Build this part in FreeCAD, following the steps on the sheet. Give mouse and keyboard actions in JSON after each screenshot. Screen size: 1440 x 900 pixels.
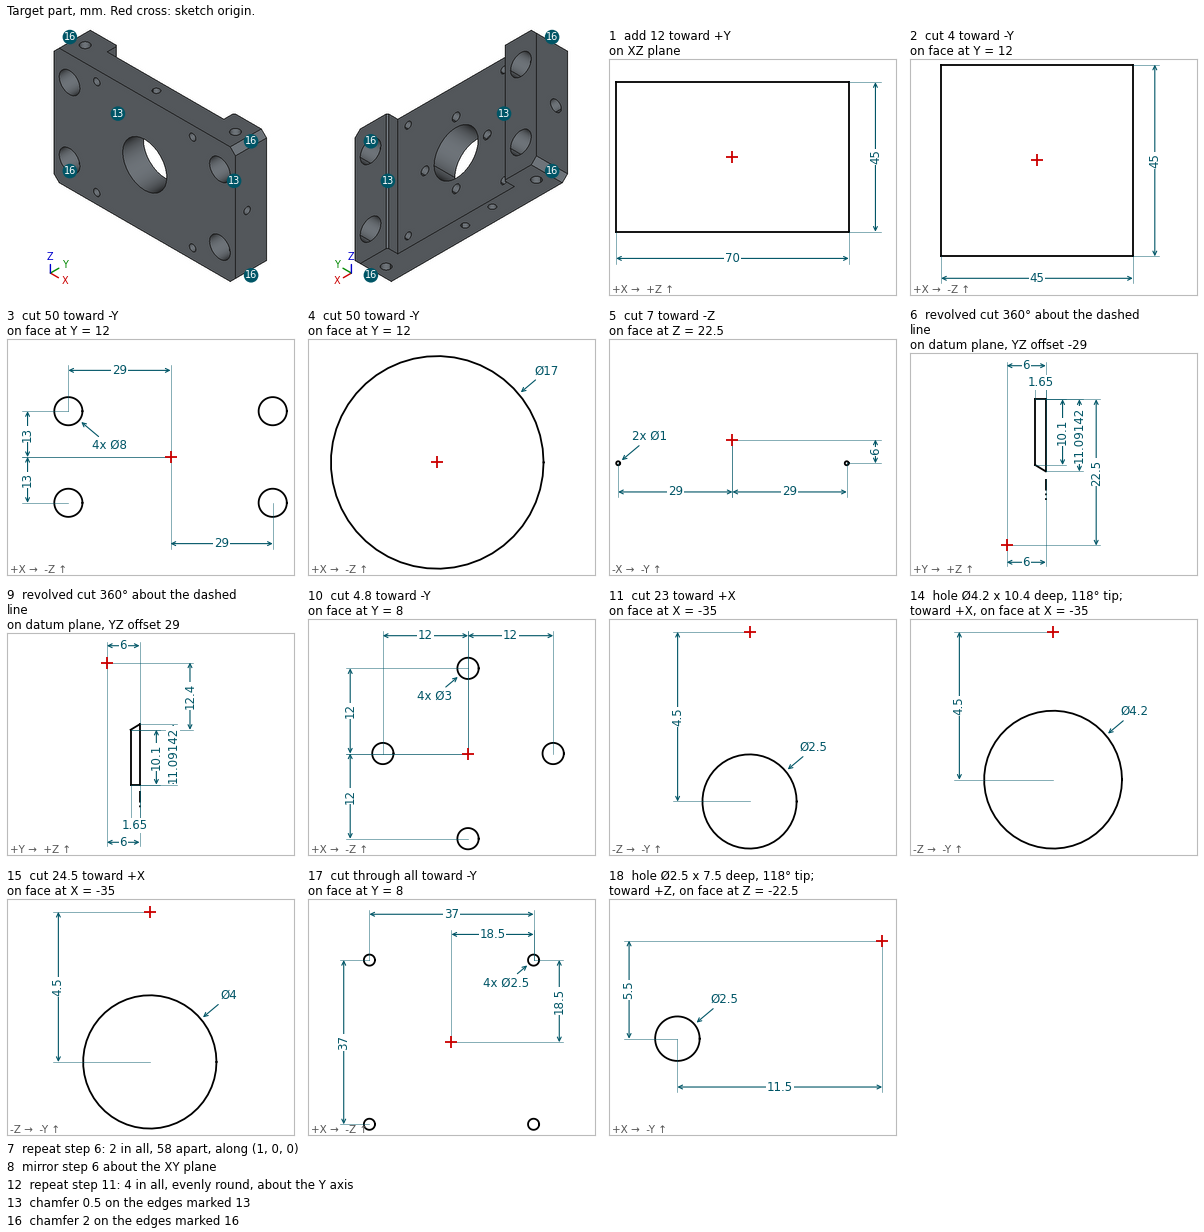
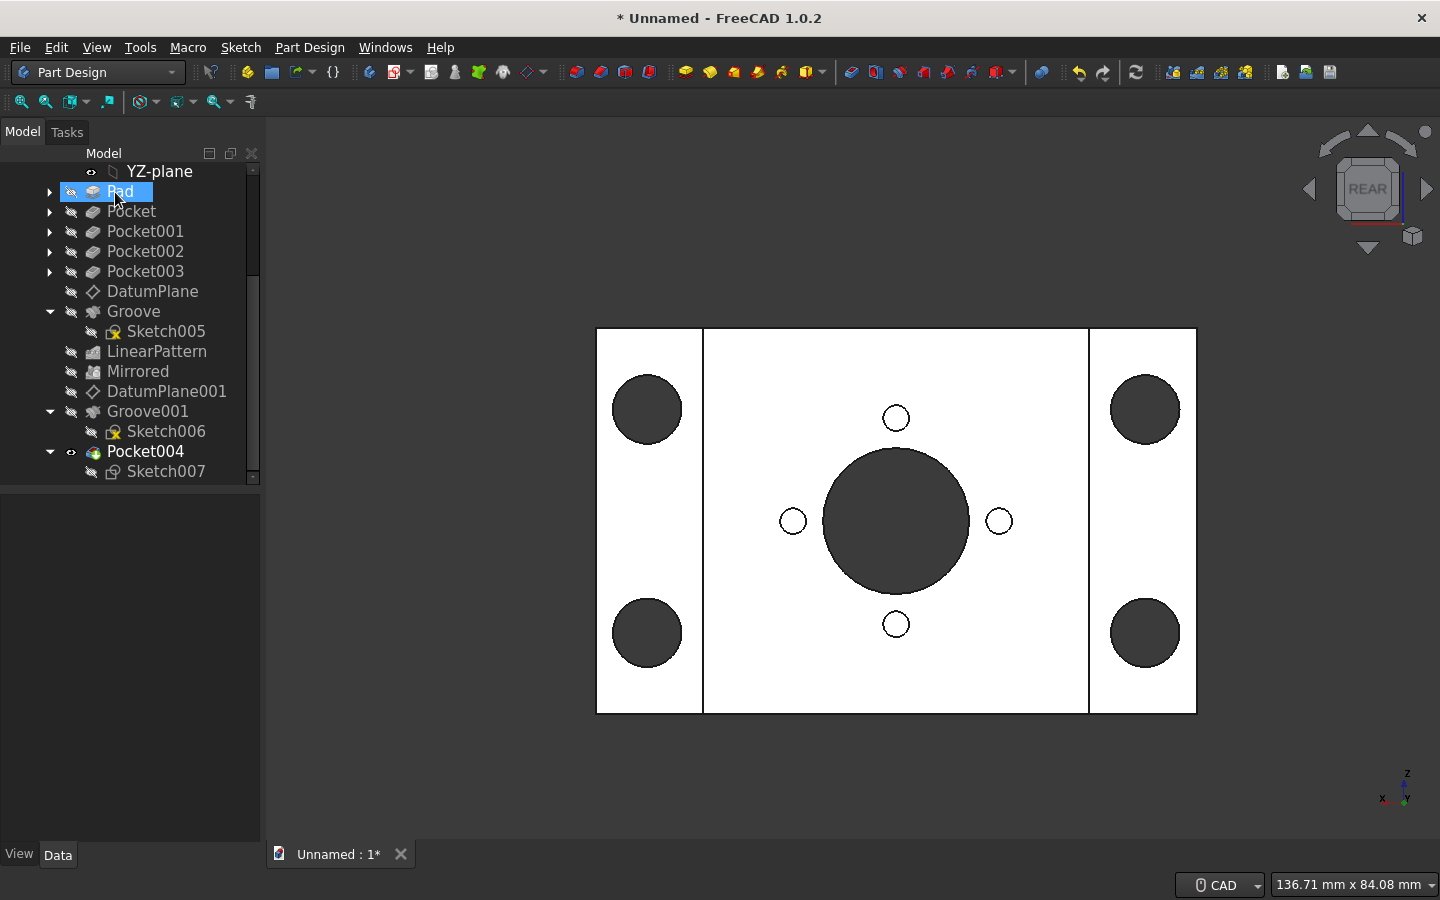
{"action": "key", "text": "6"}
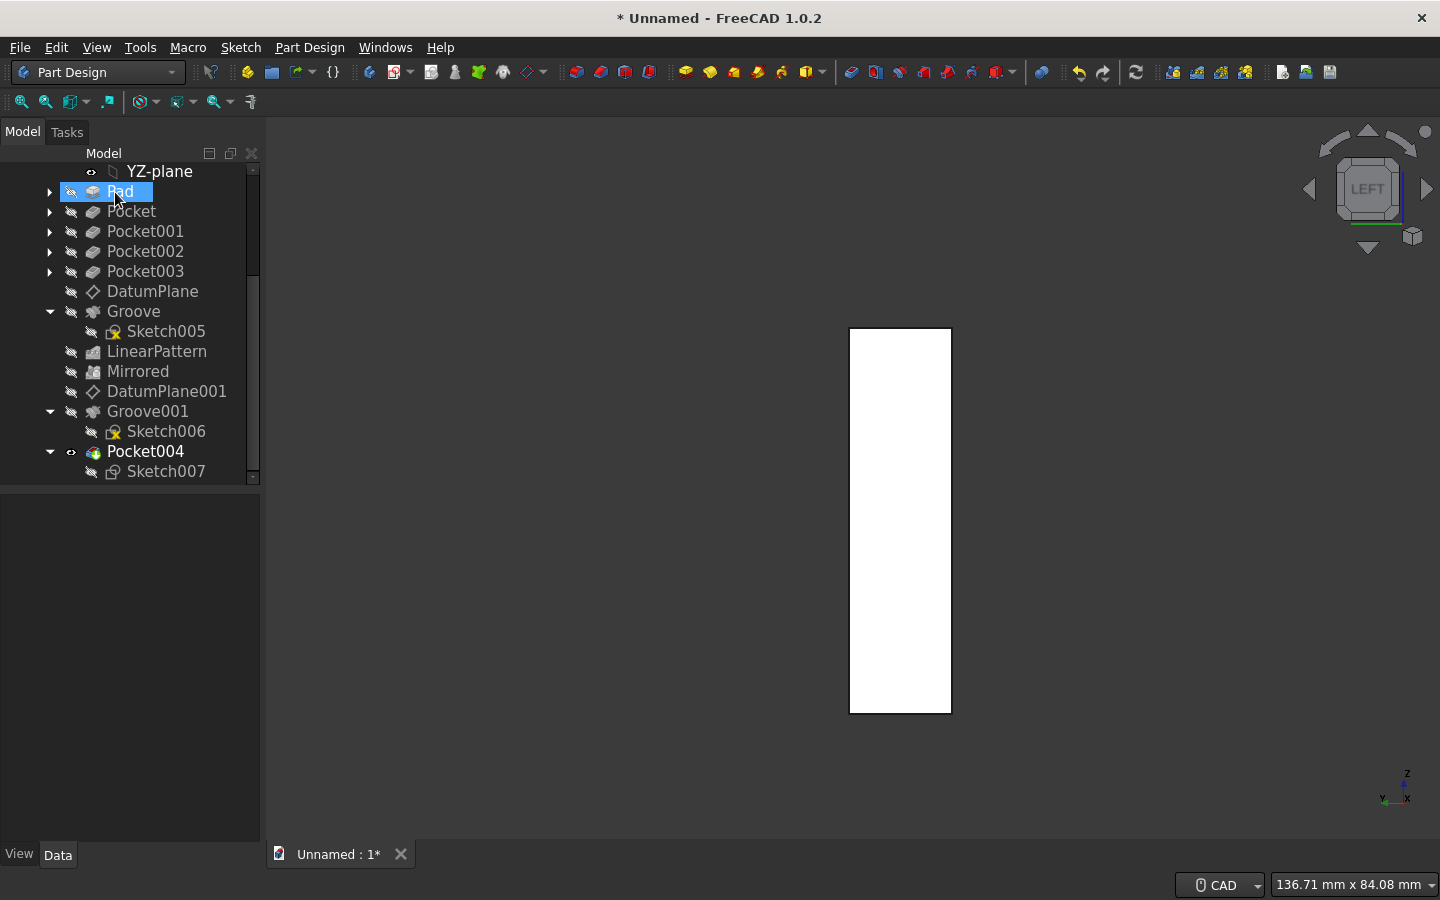
{"action": "left_click", "coordinate": [900, 410]}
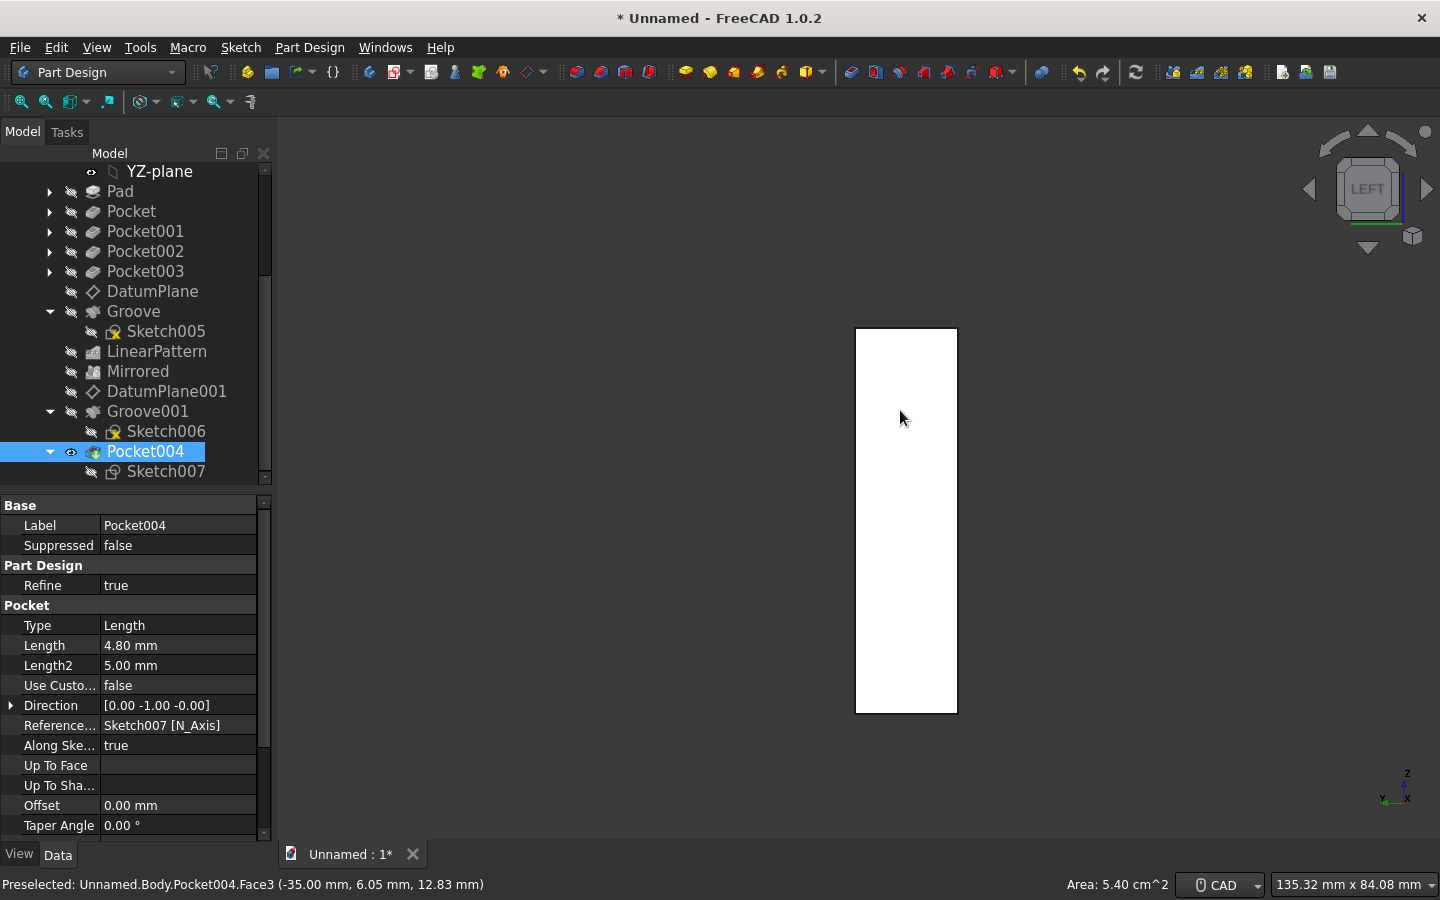
{"action": "left_click", "coordinate": [394, 72]}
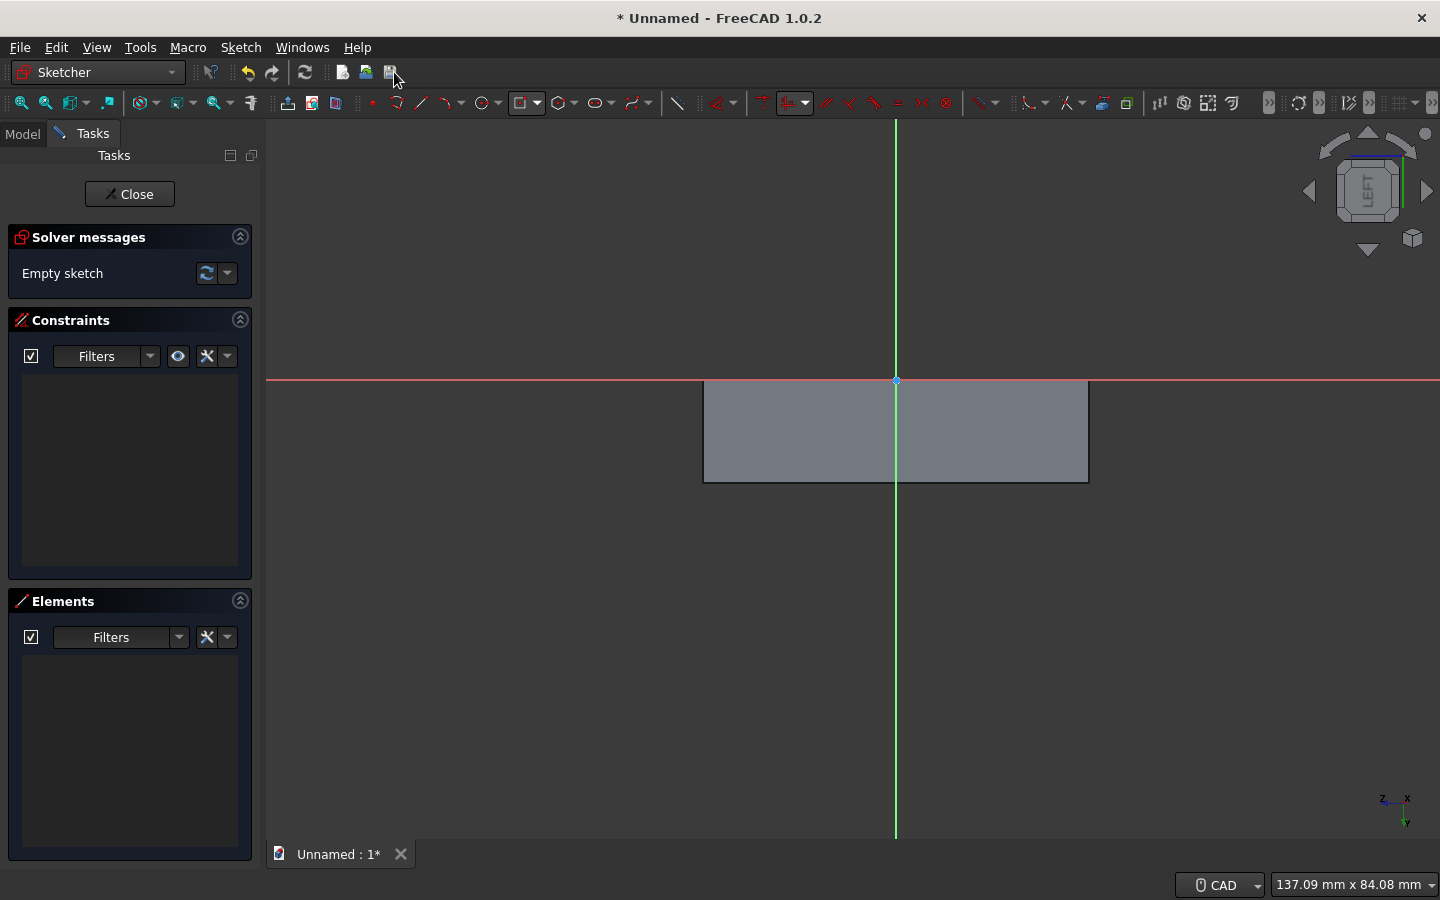
{"action": "scroll", "coordinate": [910, 396], "scroll_direction": "up", "scroll_amount": 11}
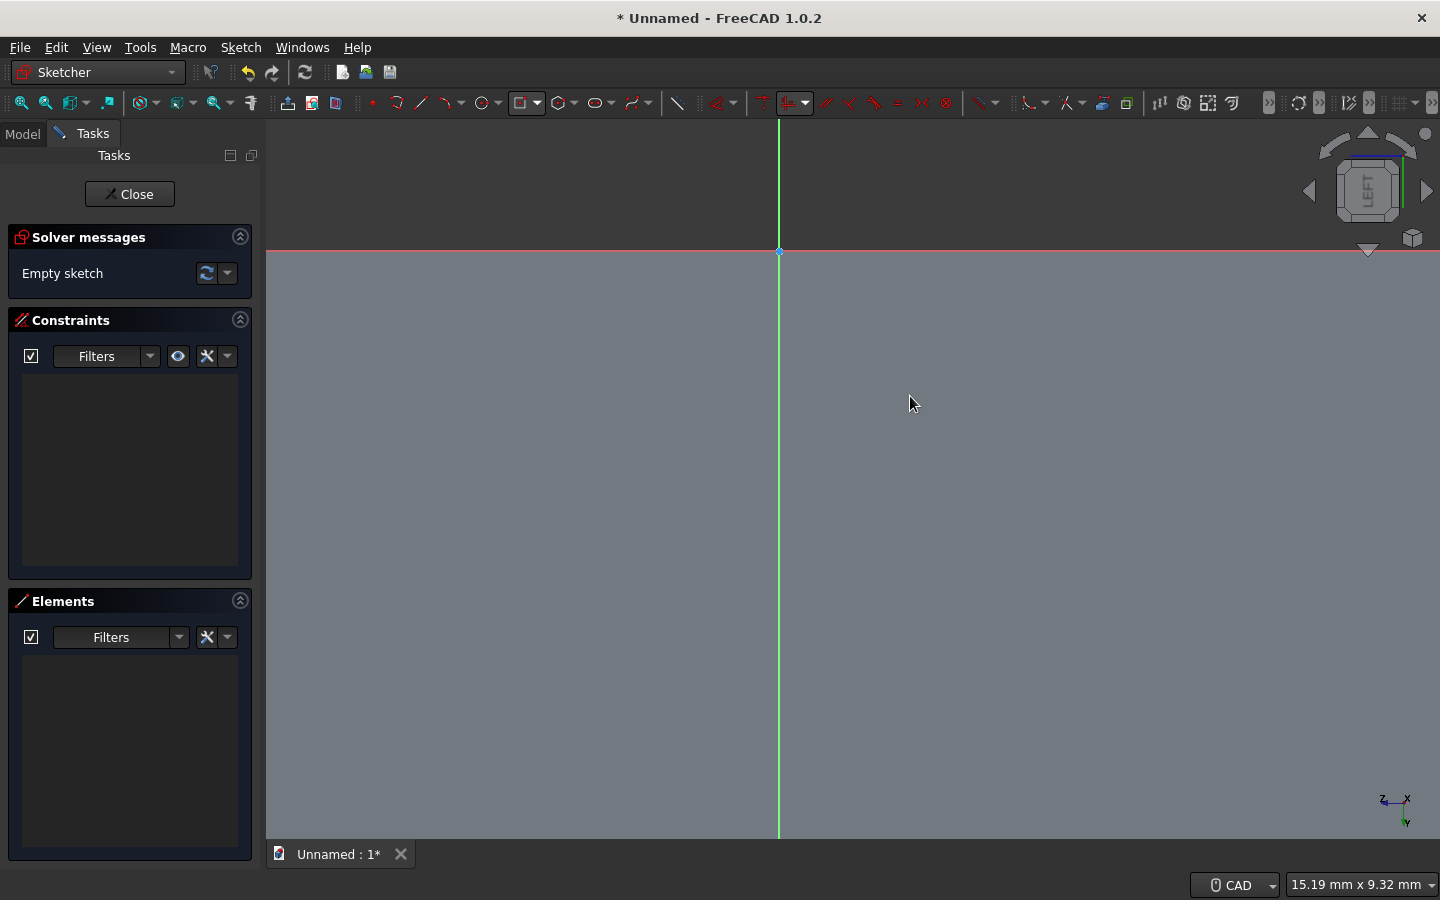
{"action": "left_click", "coordinate": [482, 104]}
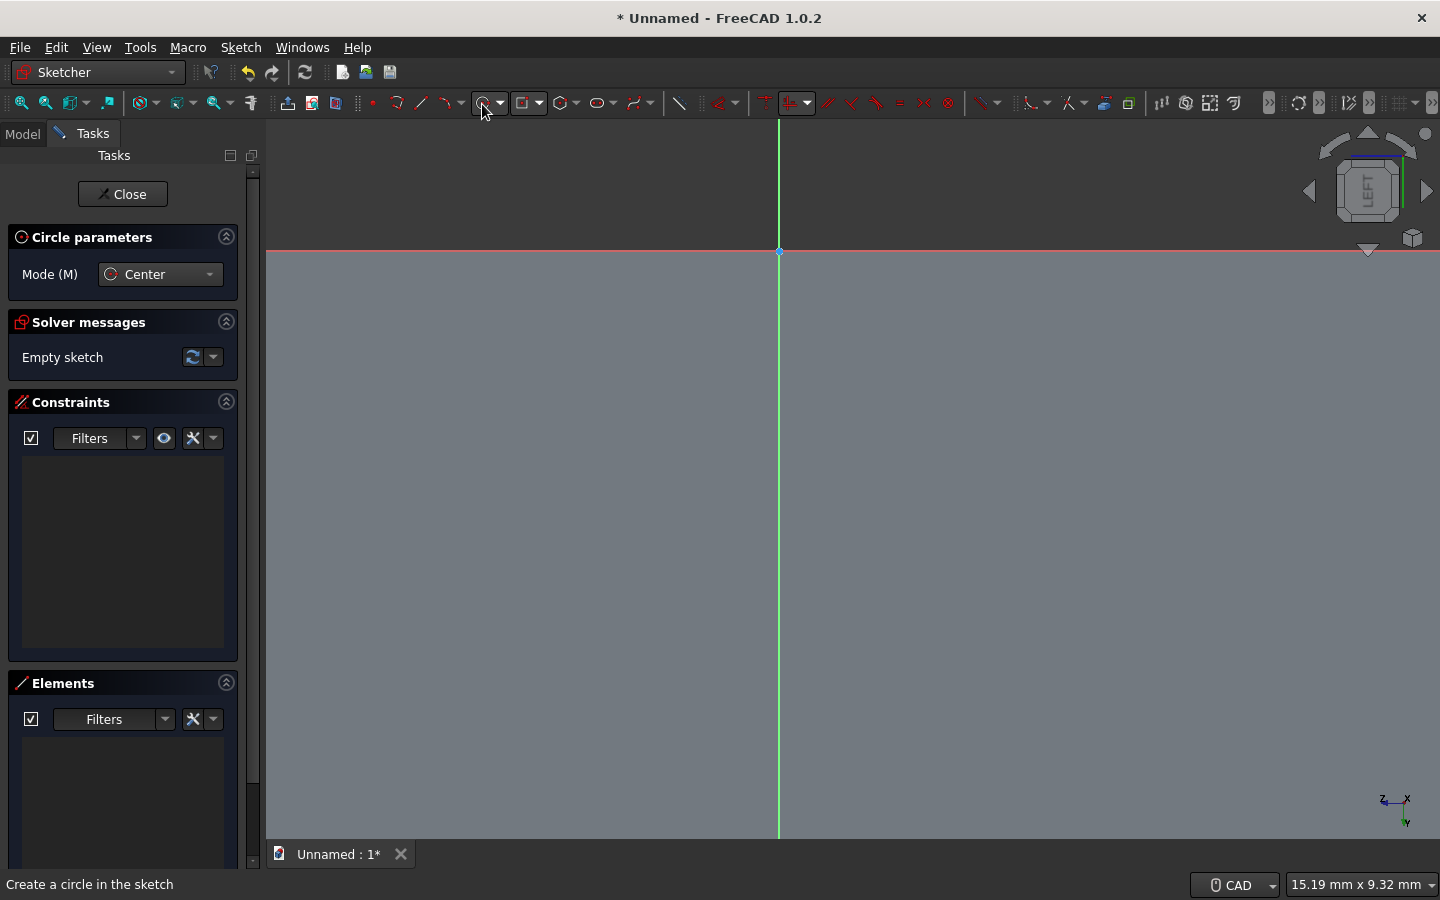
{"action": "left_click", "coordinate": [779, 599]}
{"action": "mouse_move", "coordinate": [848, 531]}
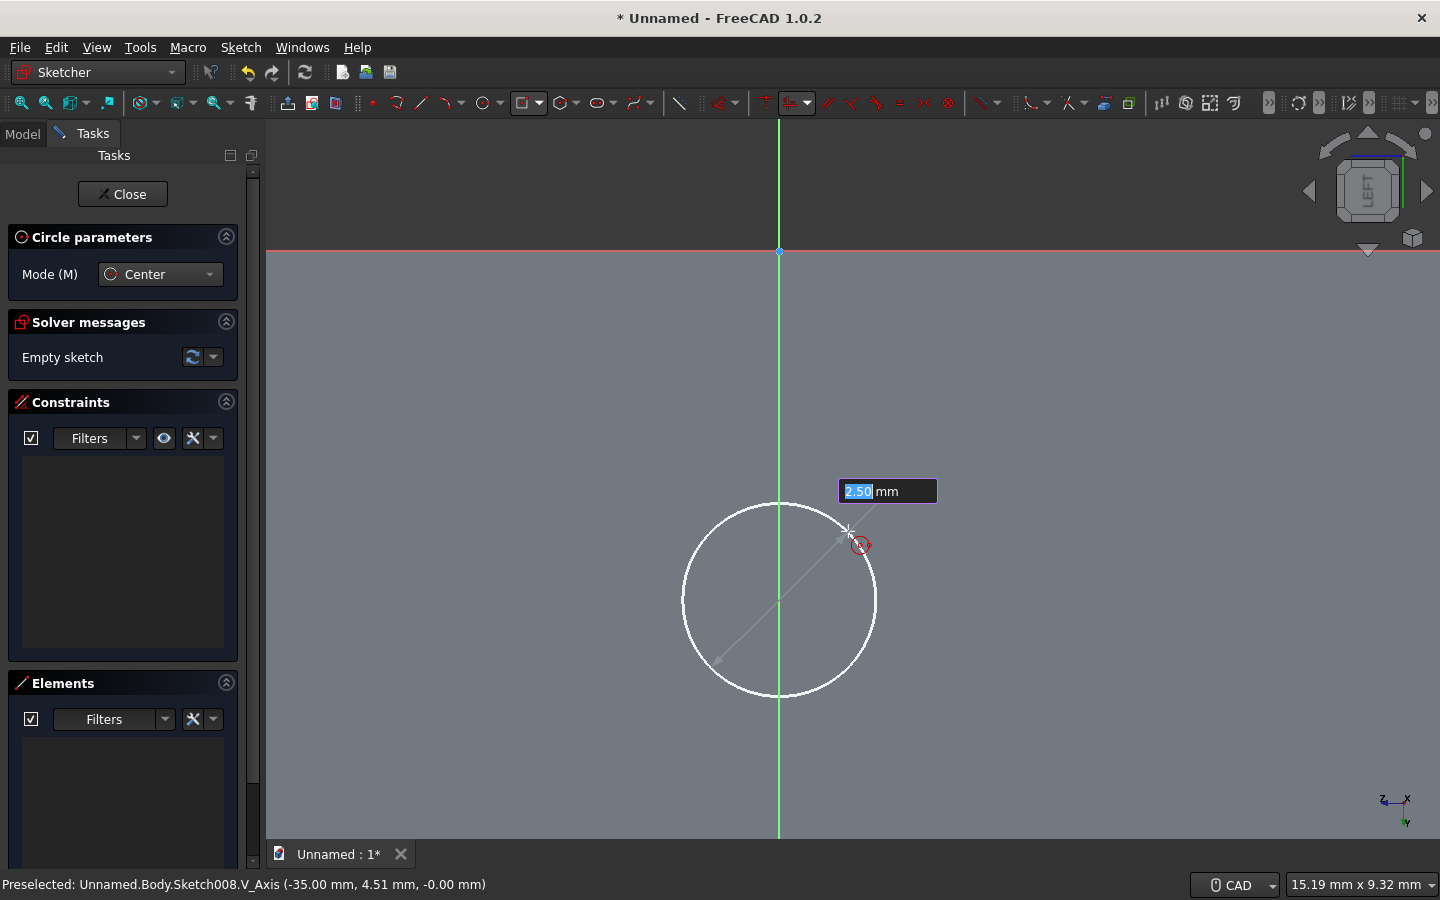
{"action": "type", "text": "2.5"}
{"action": "key", "text": "Return"}
{"action": "key", "text": "Escape"}